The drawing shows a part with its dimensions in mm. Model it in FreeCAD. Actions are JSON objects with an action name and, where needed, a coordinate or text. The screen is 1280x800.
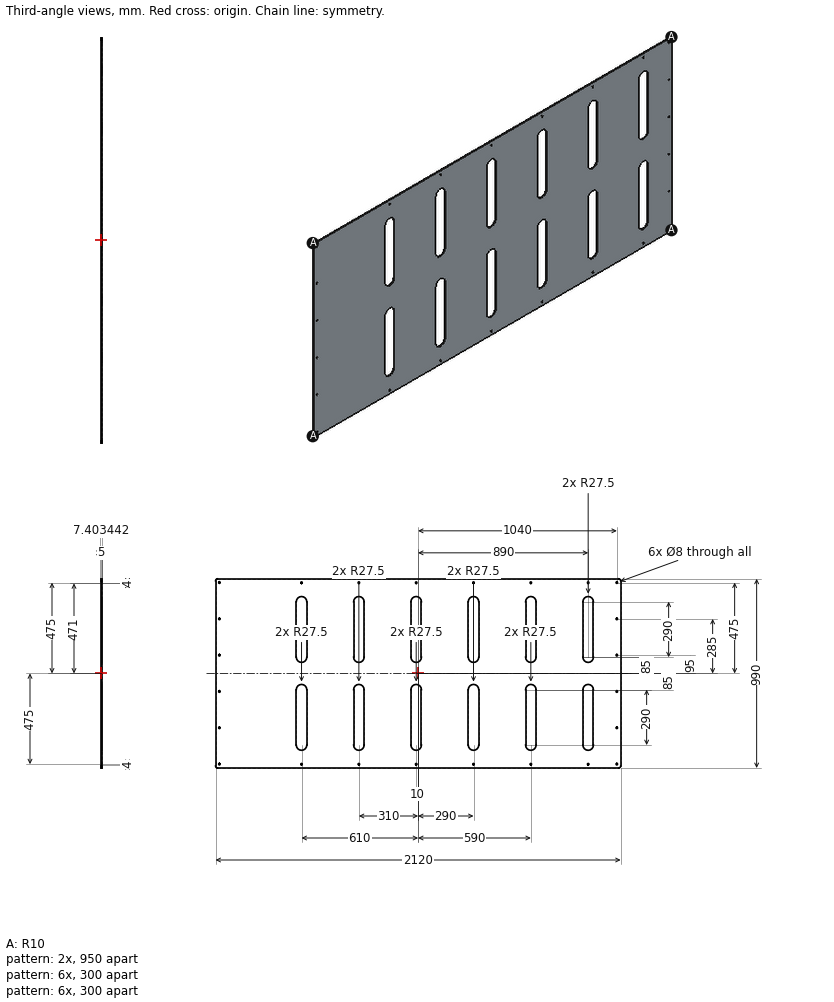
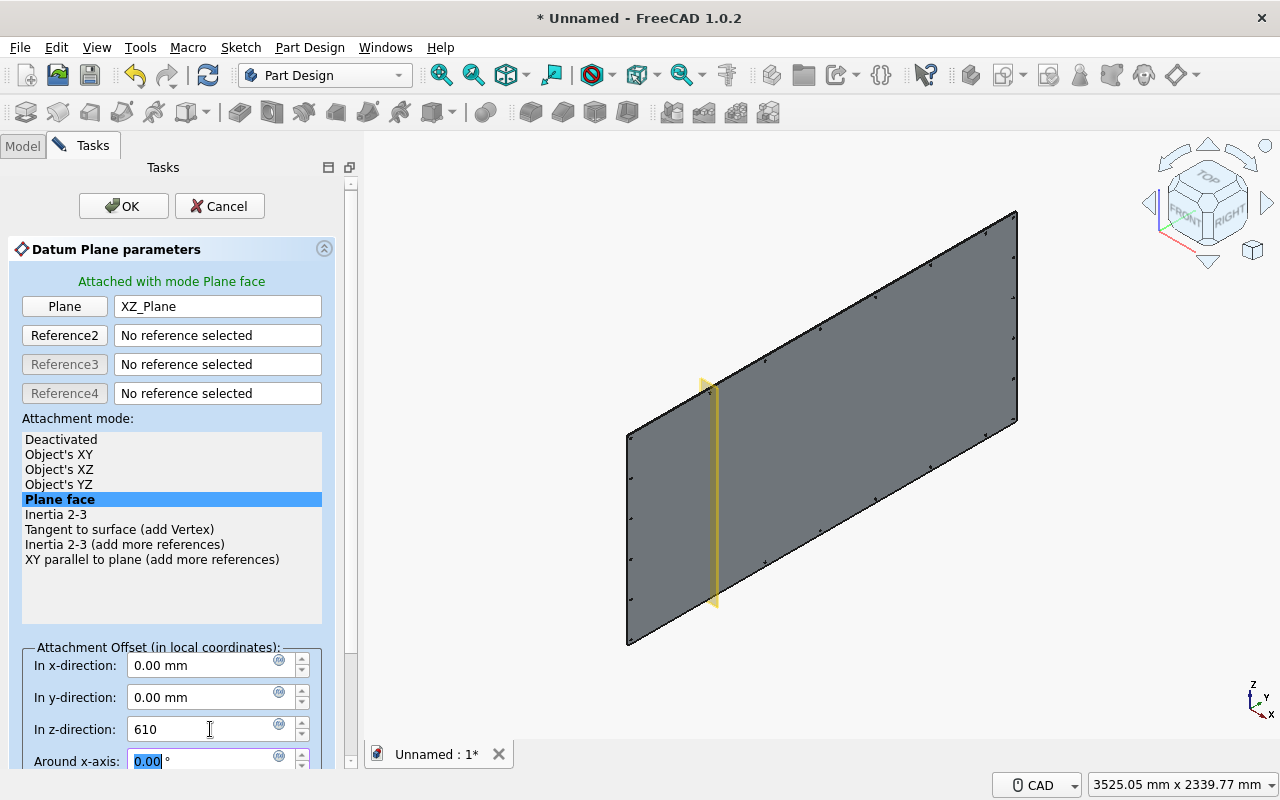
{"action": "left_click", "coordinate": [124, 206]}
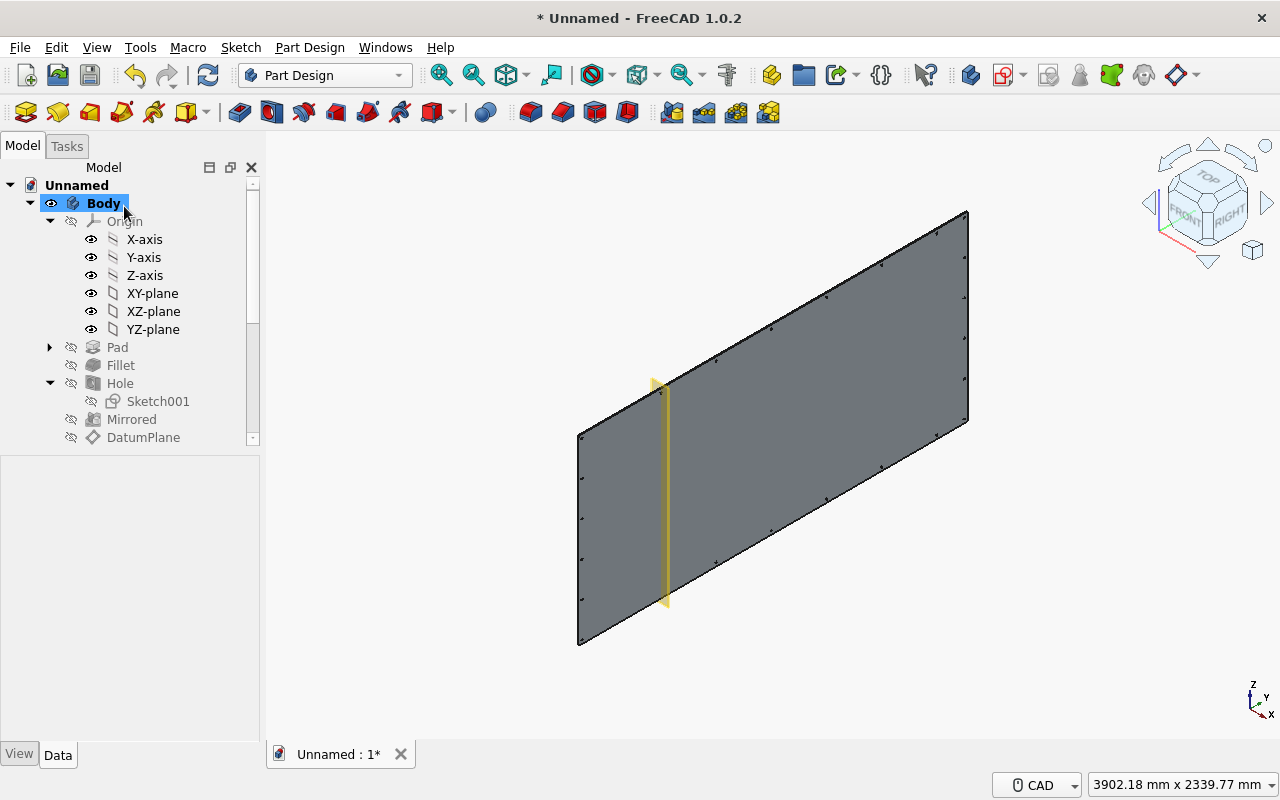
{"action": "scroll", "coordinate": [100, 307], "scroll_direction": "down", "scroll_amount": 3}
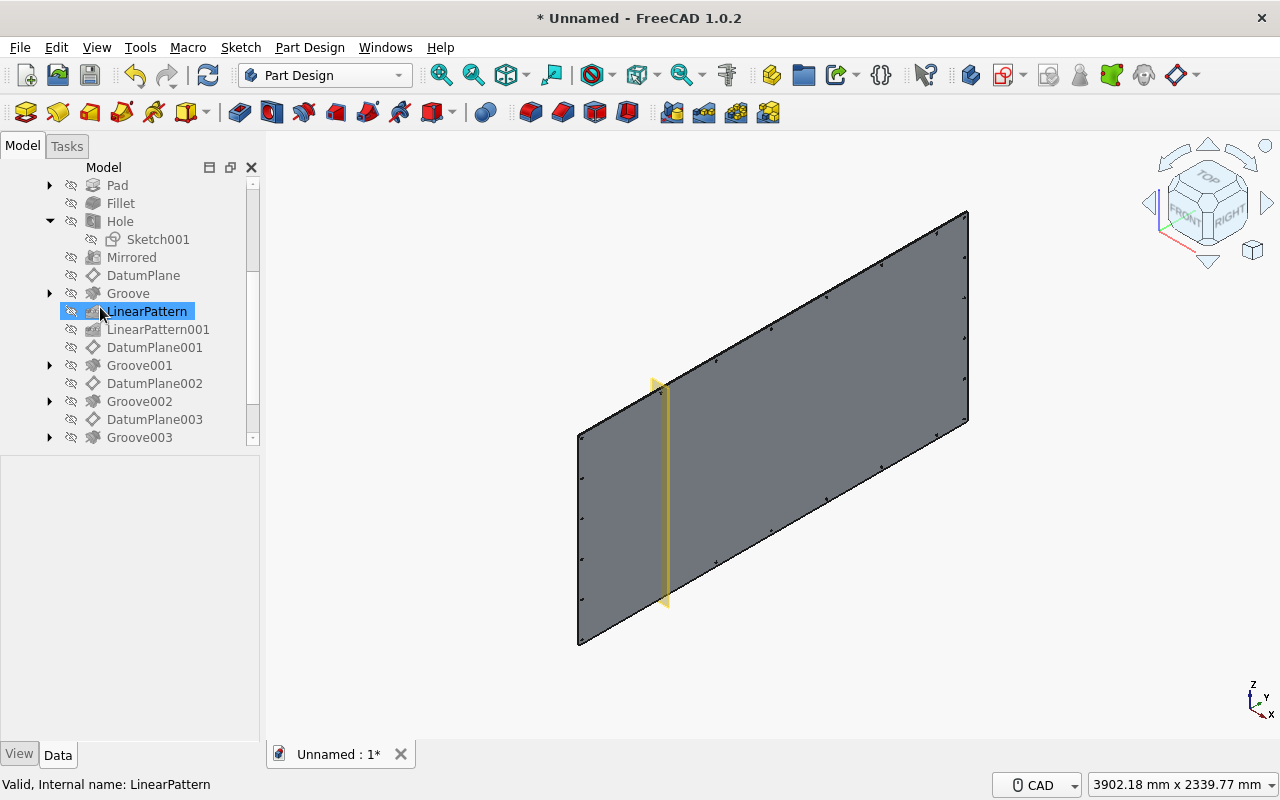
{"action": "scroll", "coordinate": [140, 307], "scroll_direction": "up", "scroll_amount": 15}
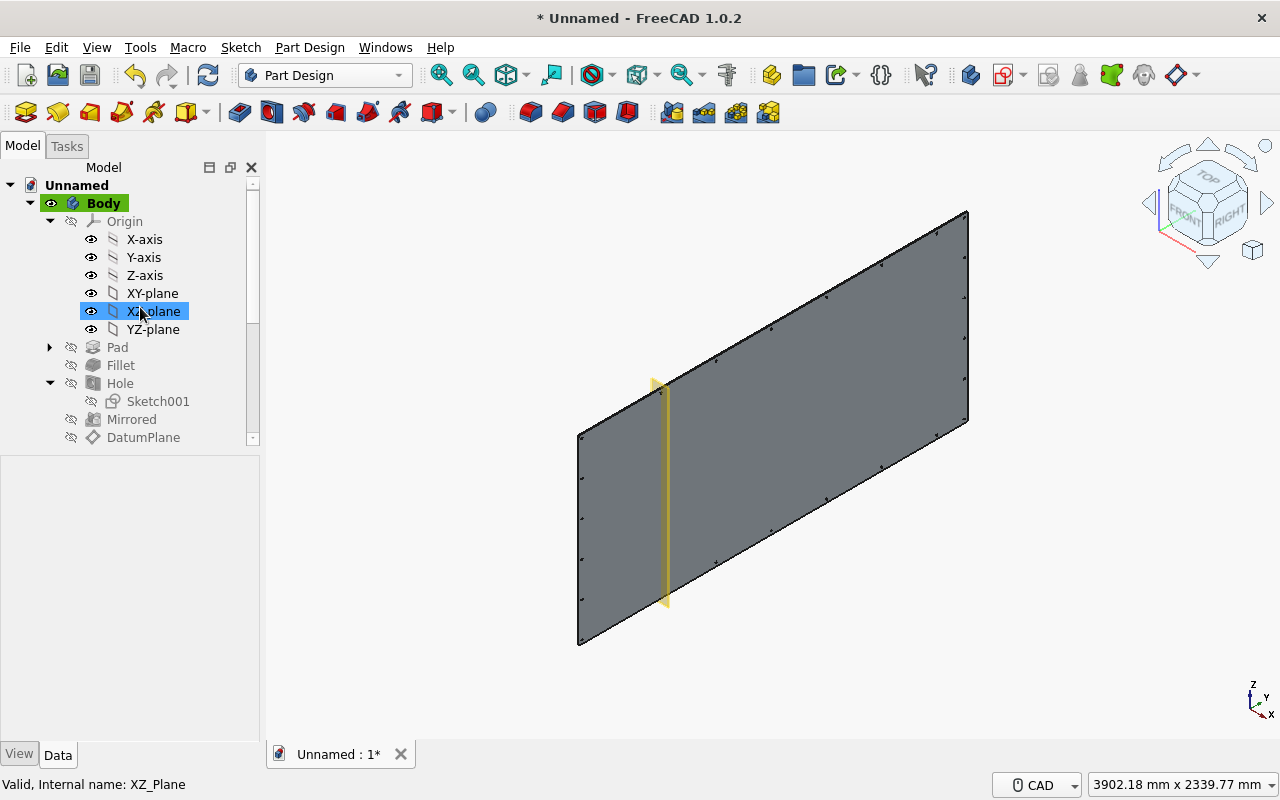
{"action": "scroll", "coordinate": [100, 307], "scroll_direction": "down", "scroll_amount": 6}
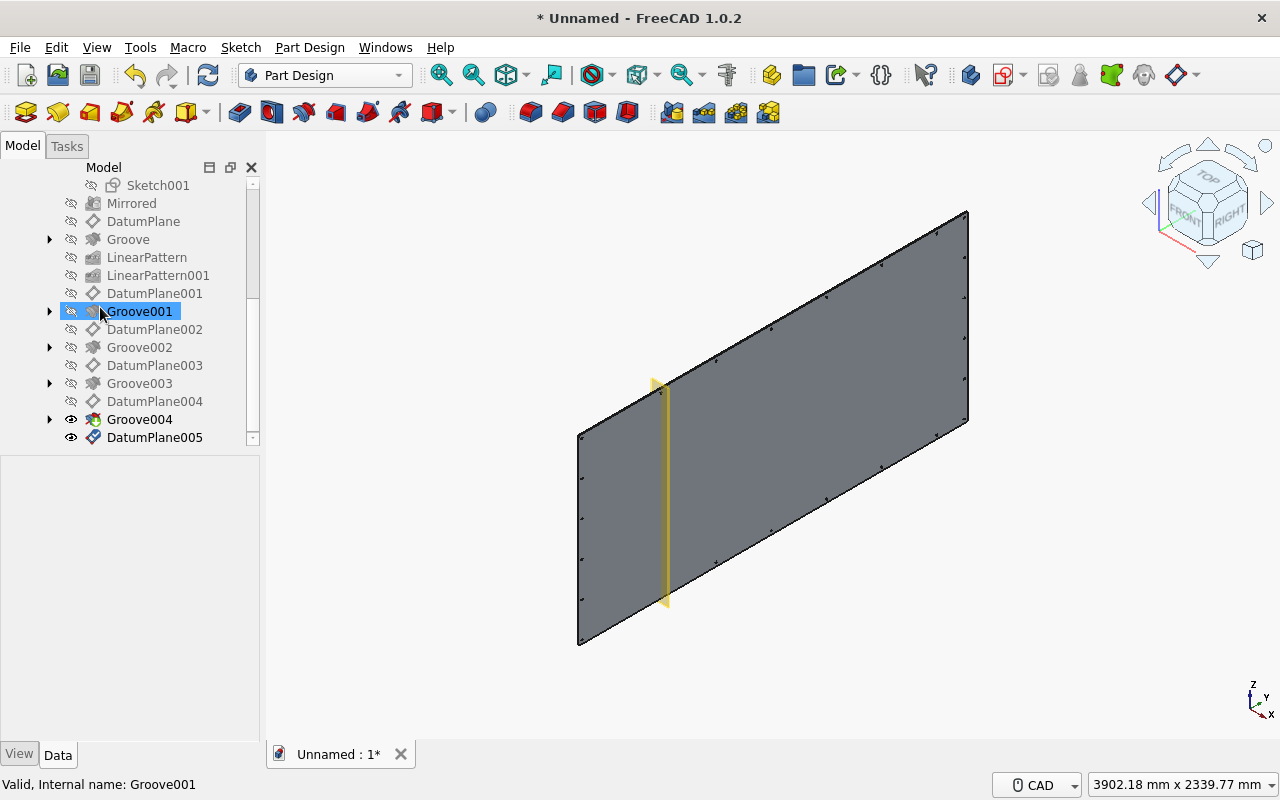
{"action": "left_click", "coordinate": [116, 437]}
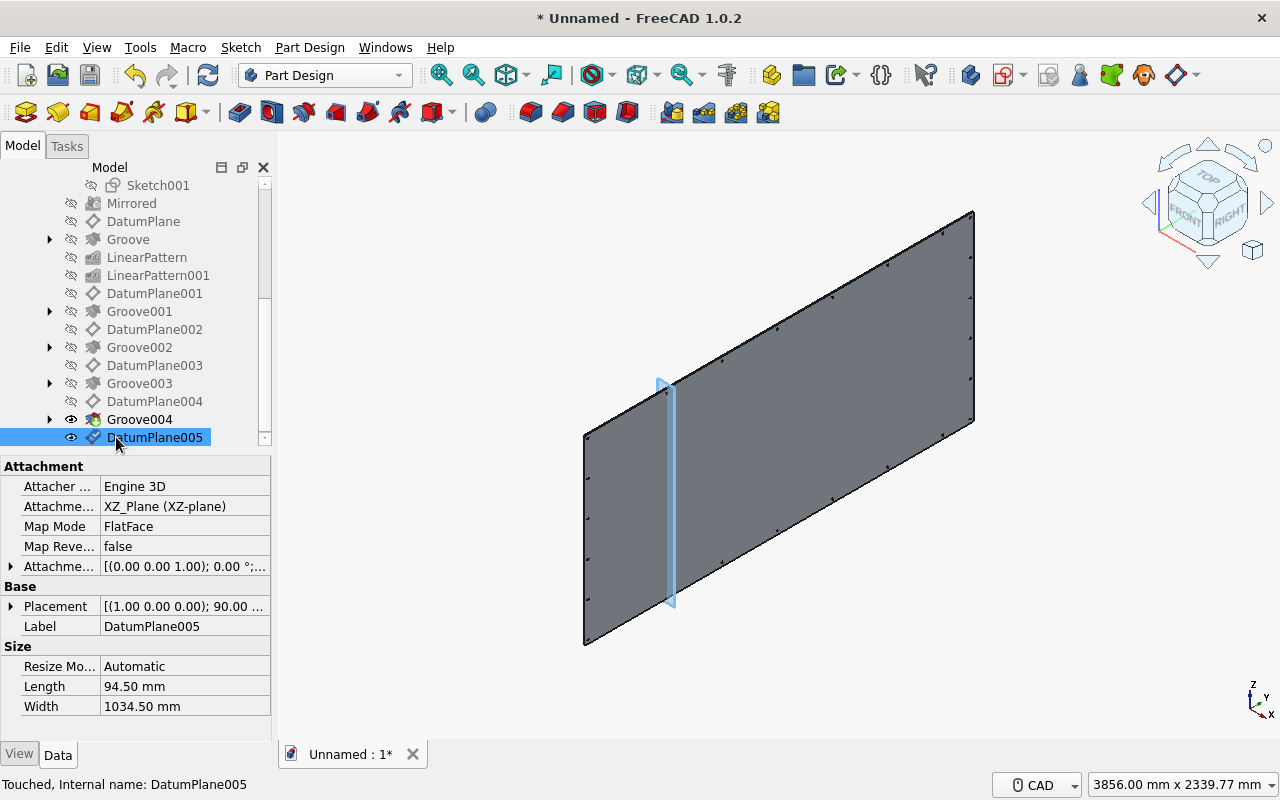
{"action": "left_click", "coordinate": [1004, 76]}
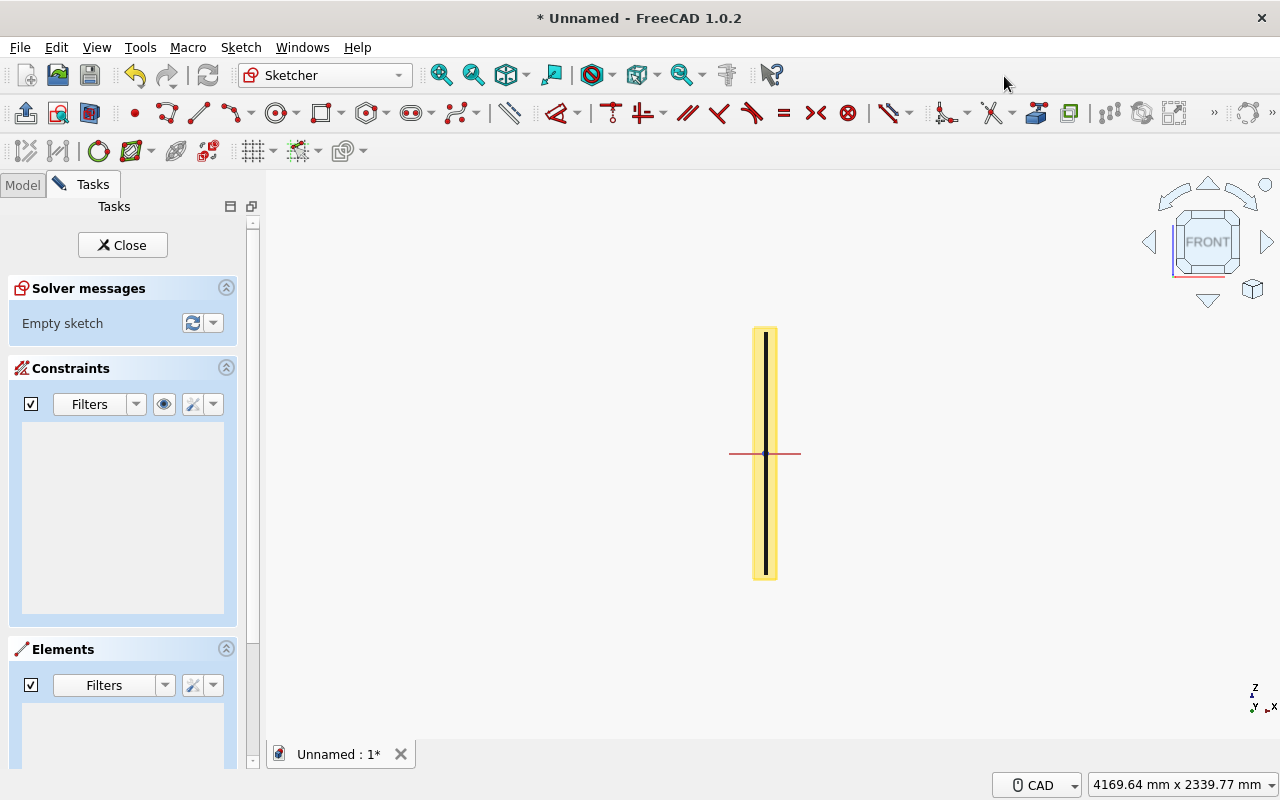
{"action": "left_click", "coordinate": [90, 114]}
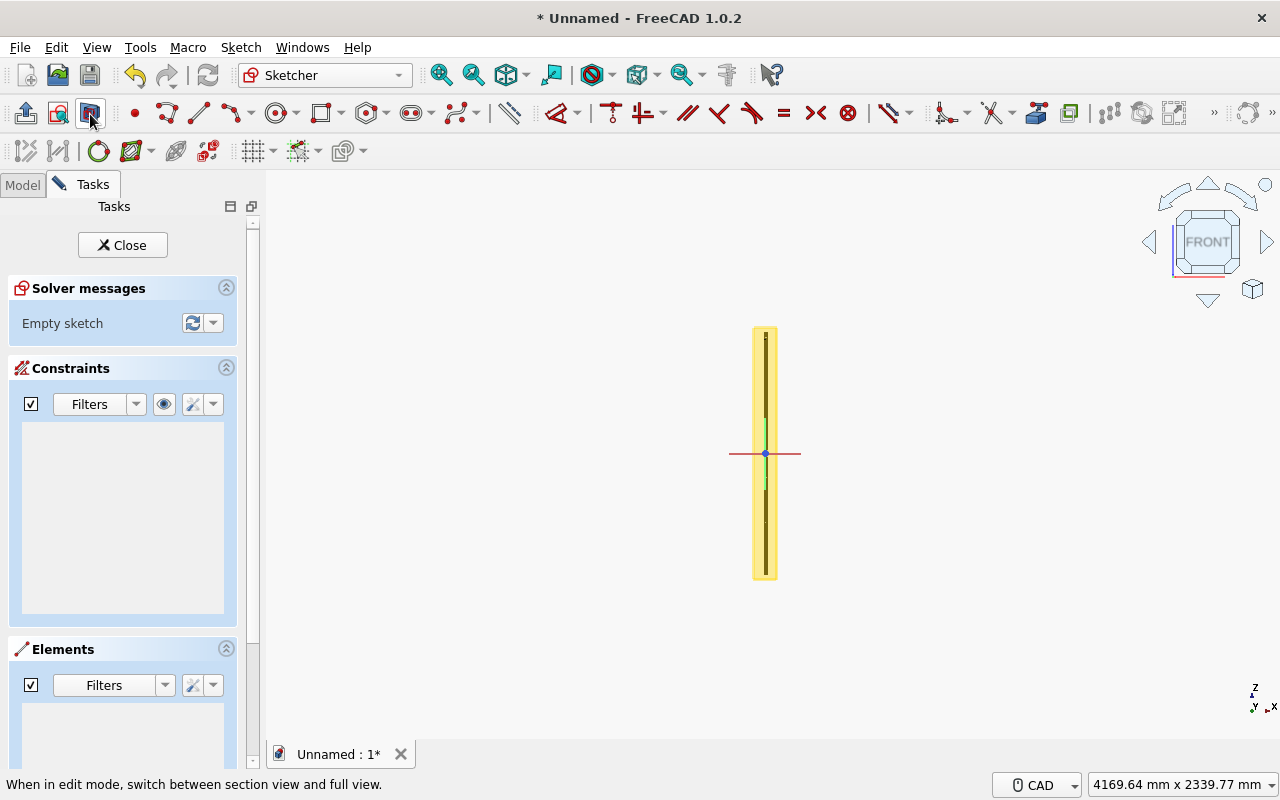
{"action": "scroll", "coordinate": [769, 576], "scroll_direction": "up", "scroll_amount": 15}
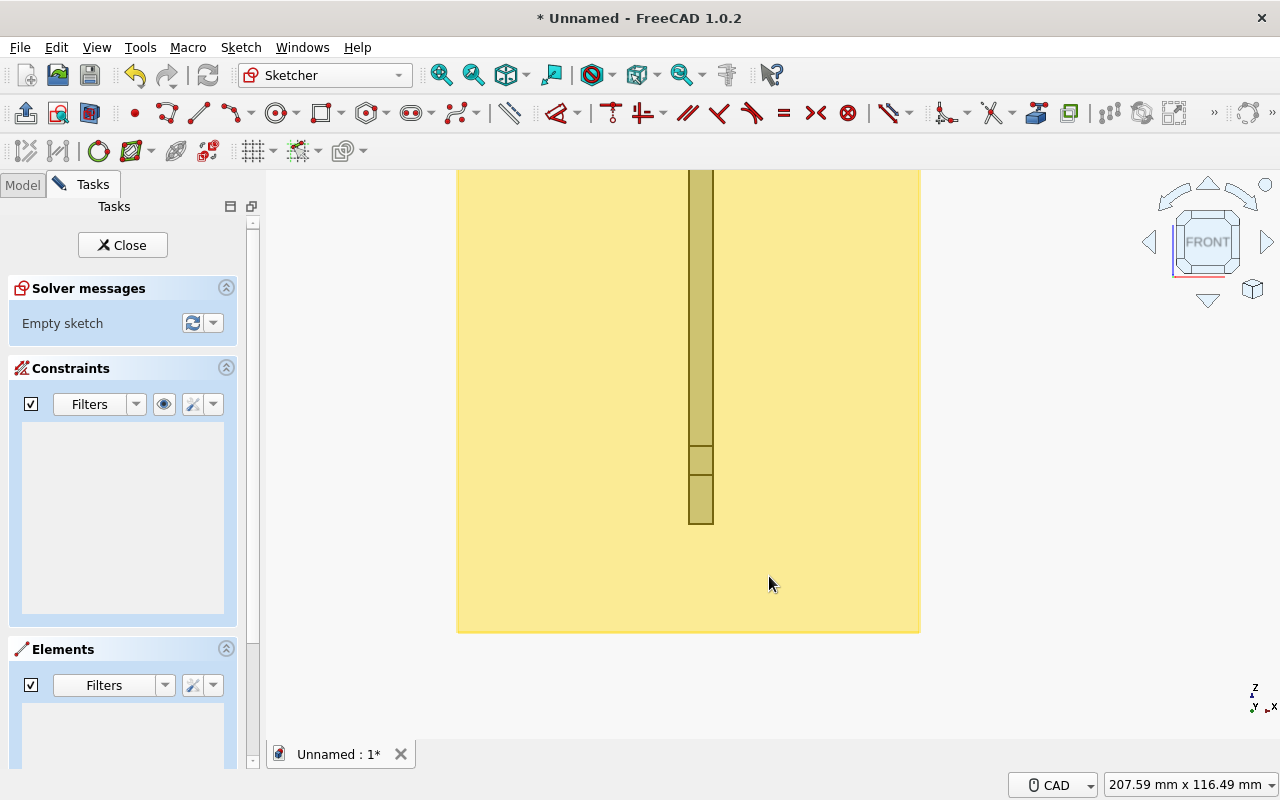
{"action": "scroll", "coordinate": [686, 434], "scroll_direction": "up", "scroll_amount": 12}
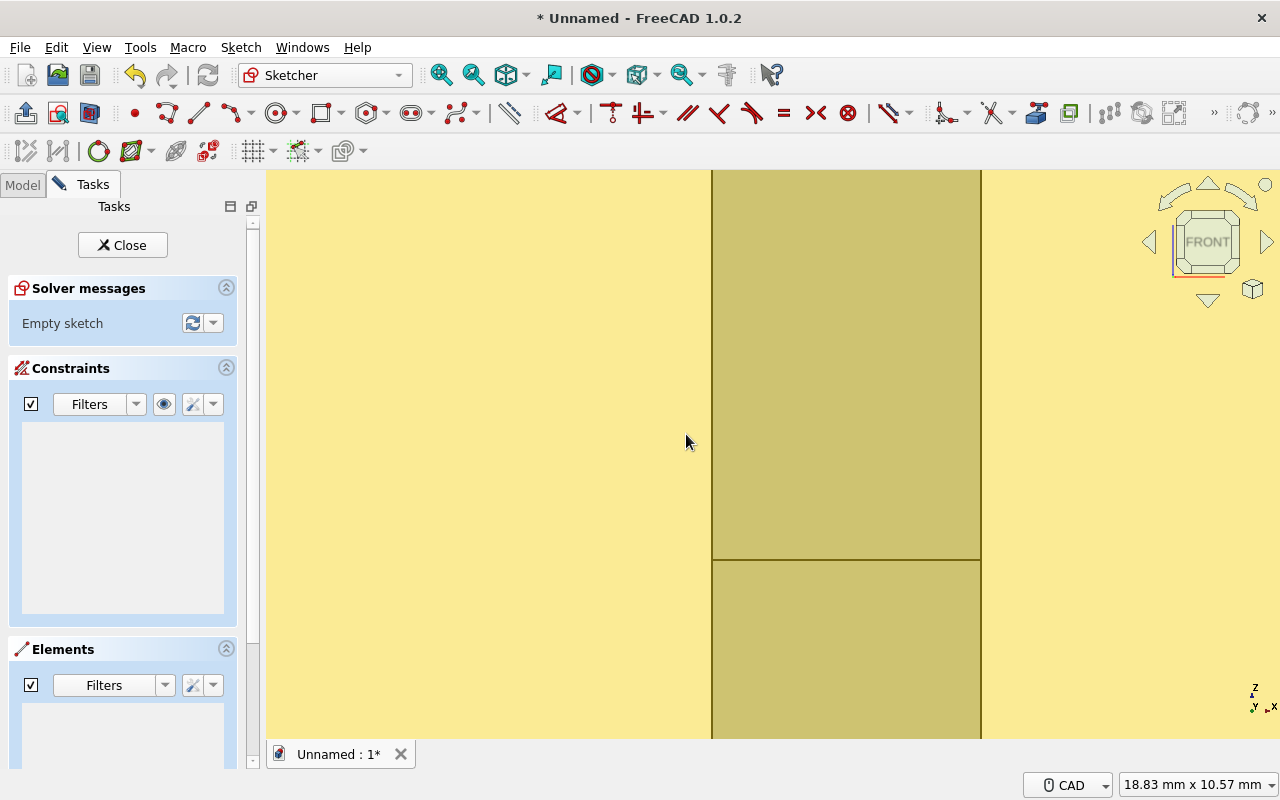
{"action": "left_click", "coordinate": [168, 114]}